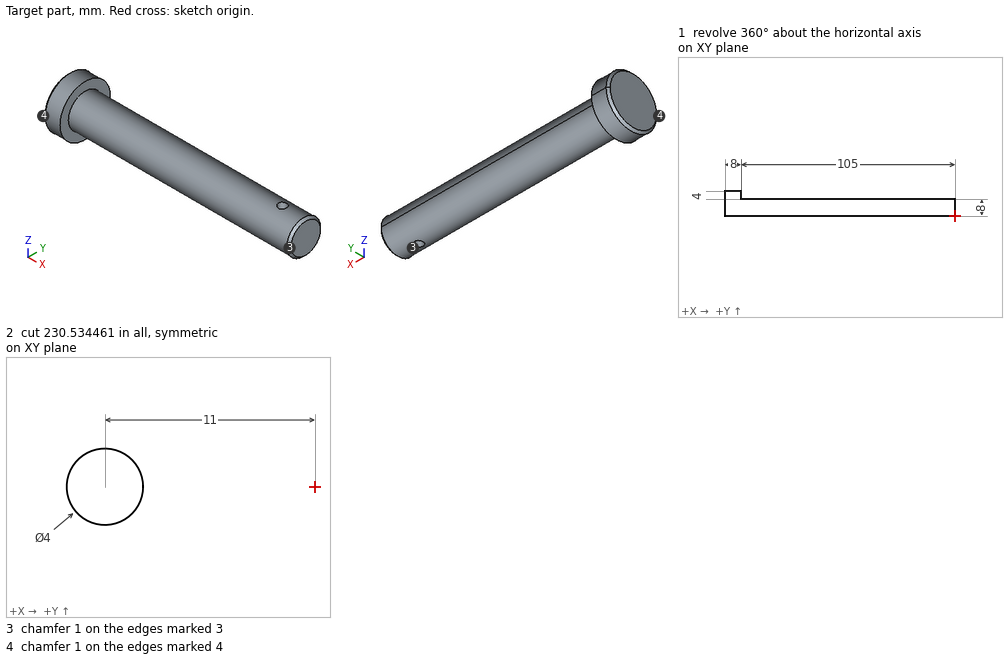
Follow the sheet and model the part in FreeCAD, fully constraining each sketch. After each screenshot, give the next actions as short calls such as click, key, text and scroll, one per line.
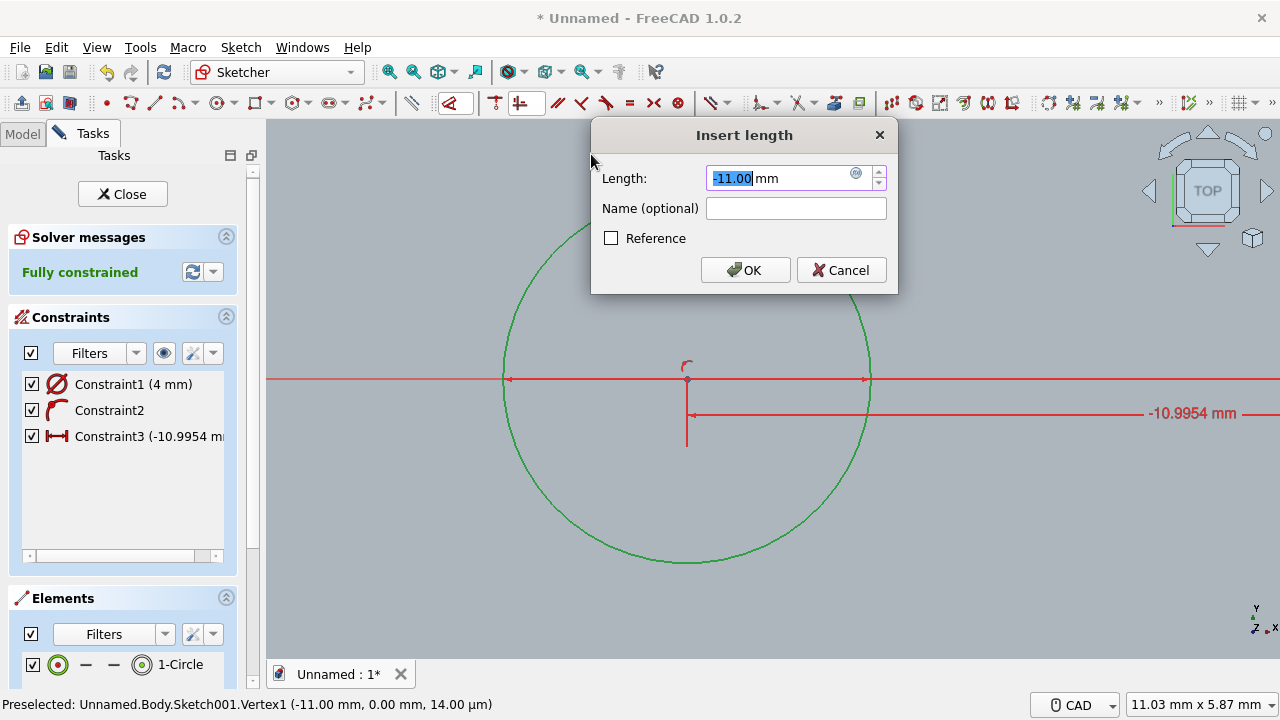
text(-11)
key(Return)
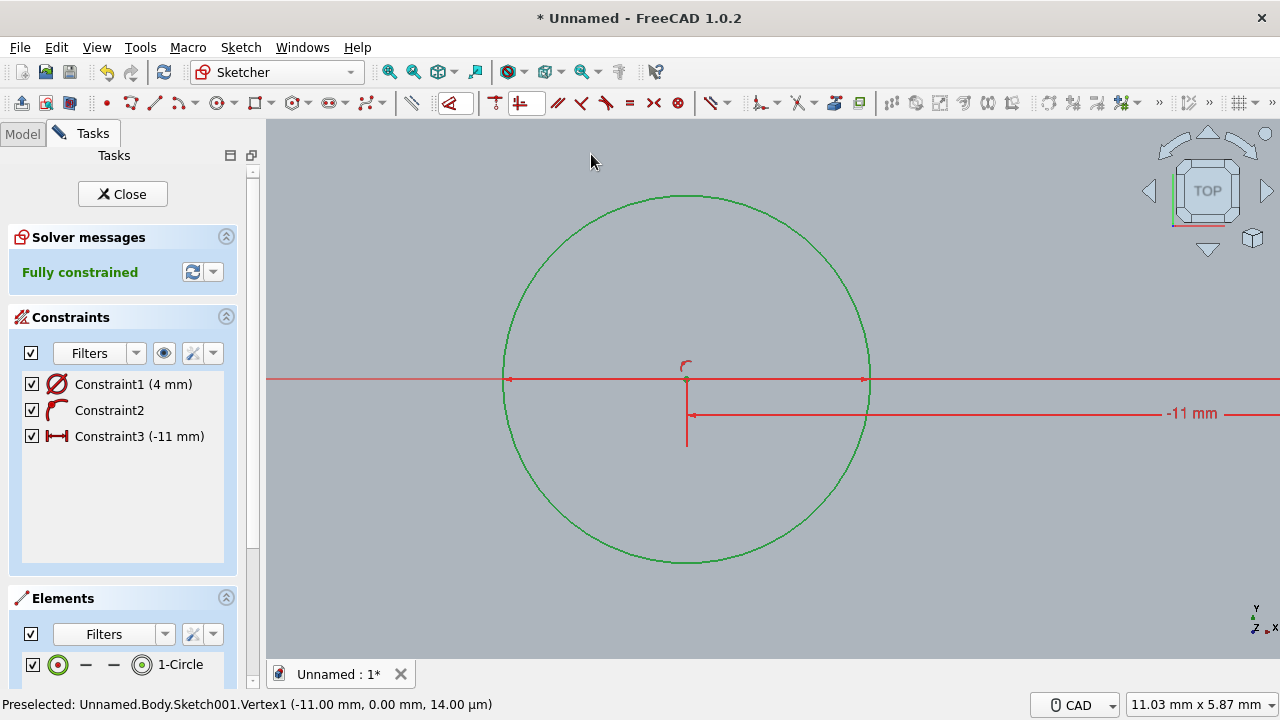
click(123, 194)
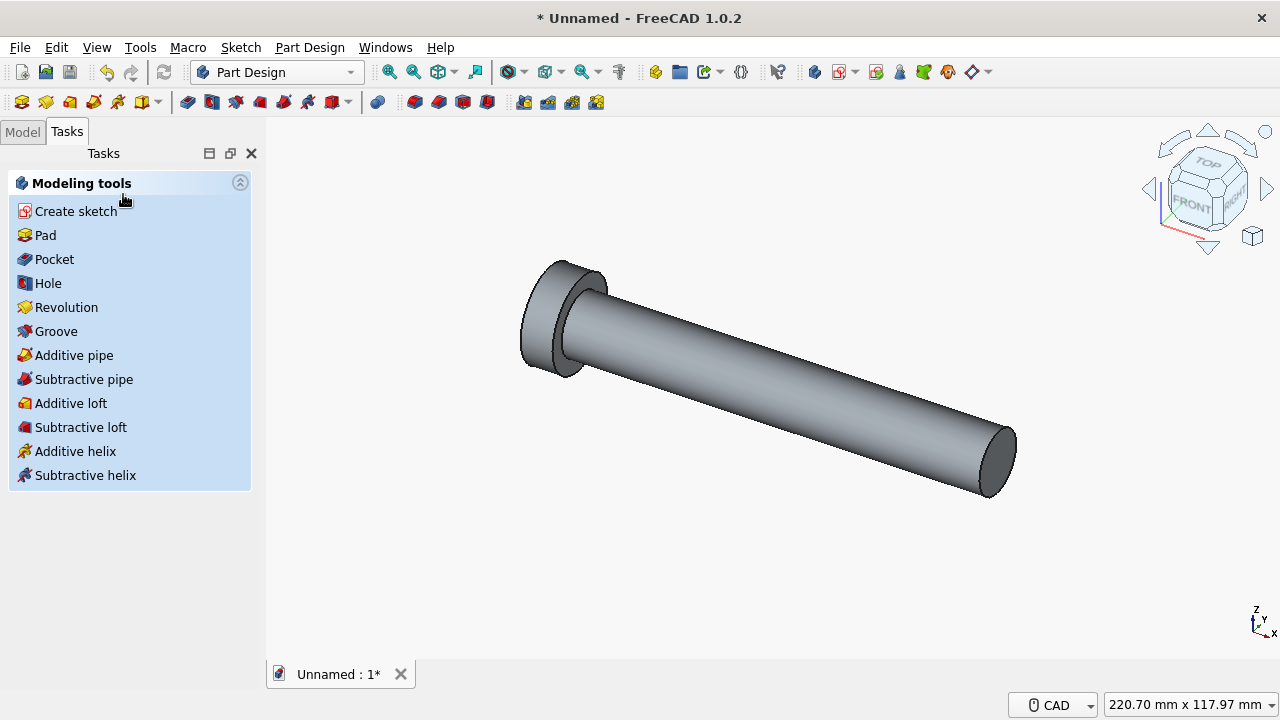
click(188, 102)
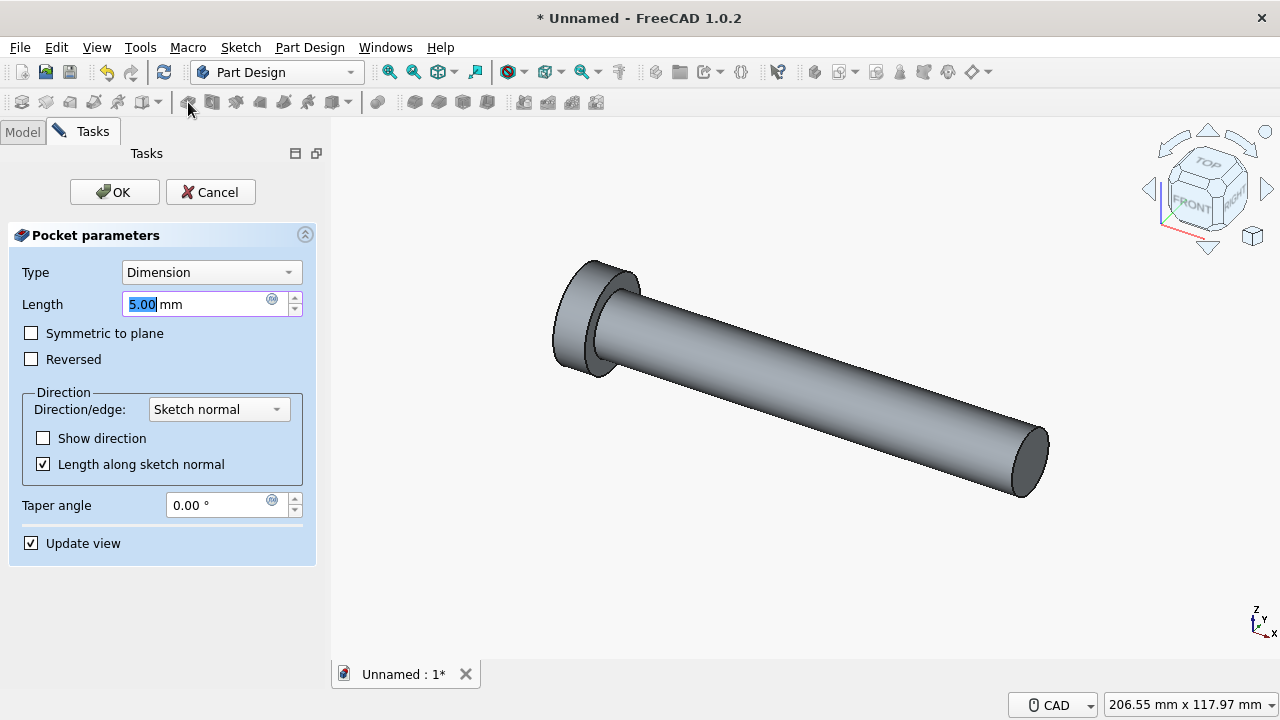
text(230.534461)
key(Tab)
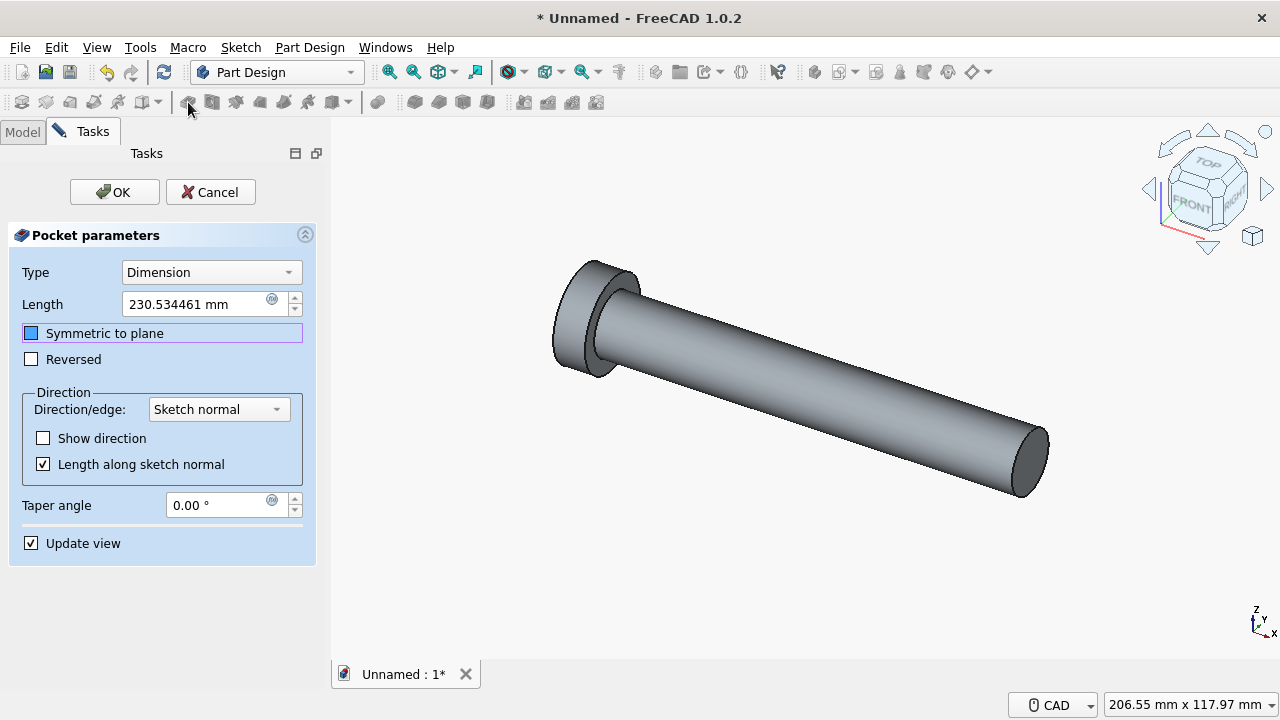
click(30, 333)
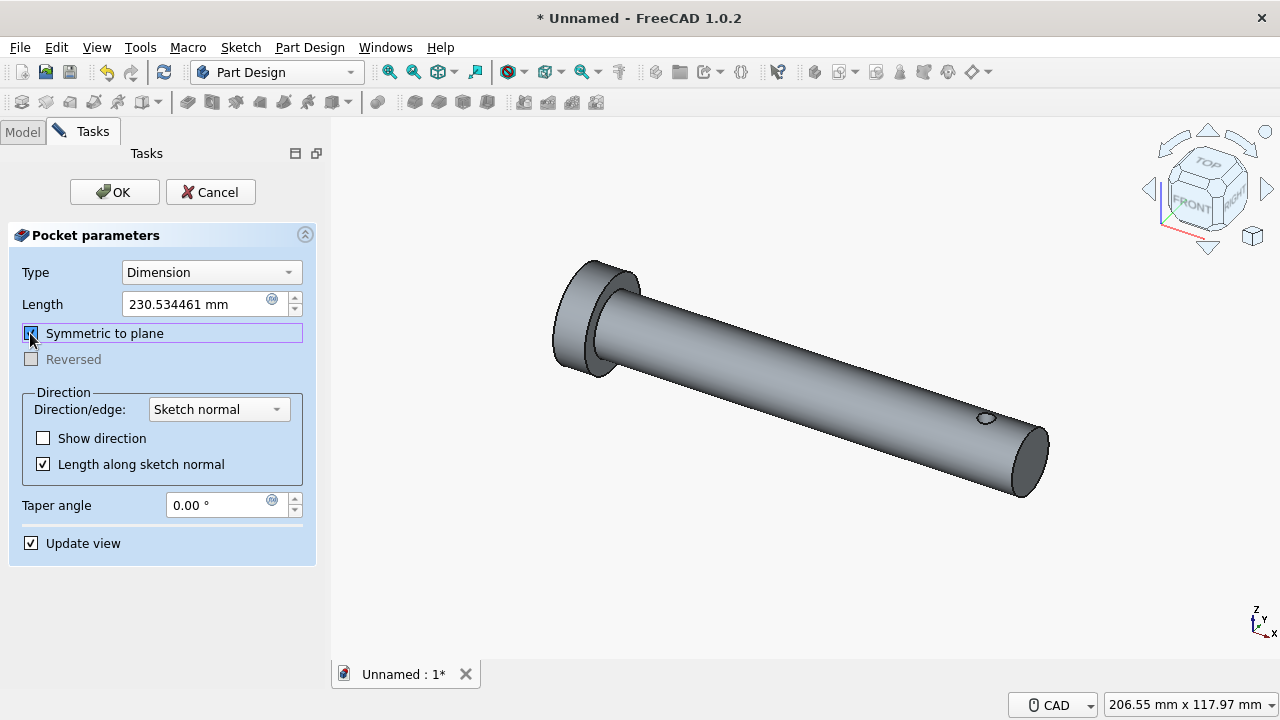
click(115, 192)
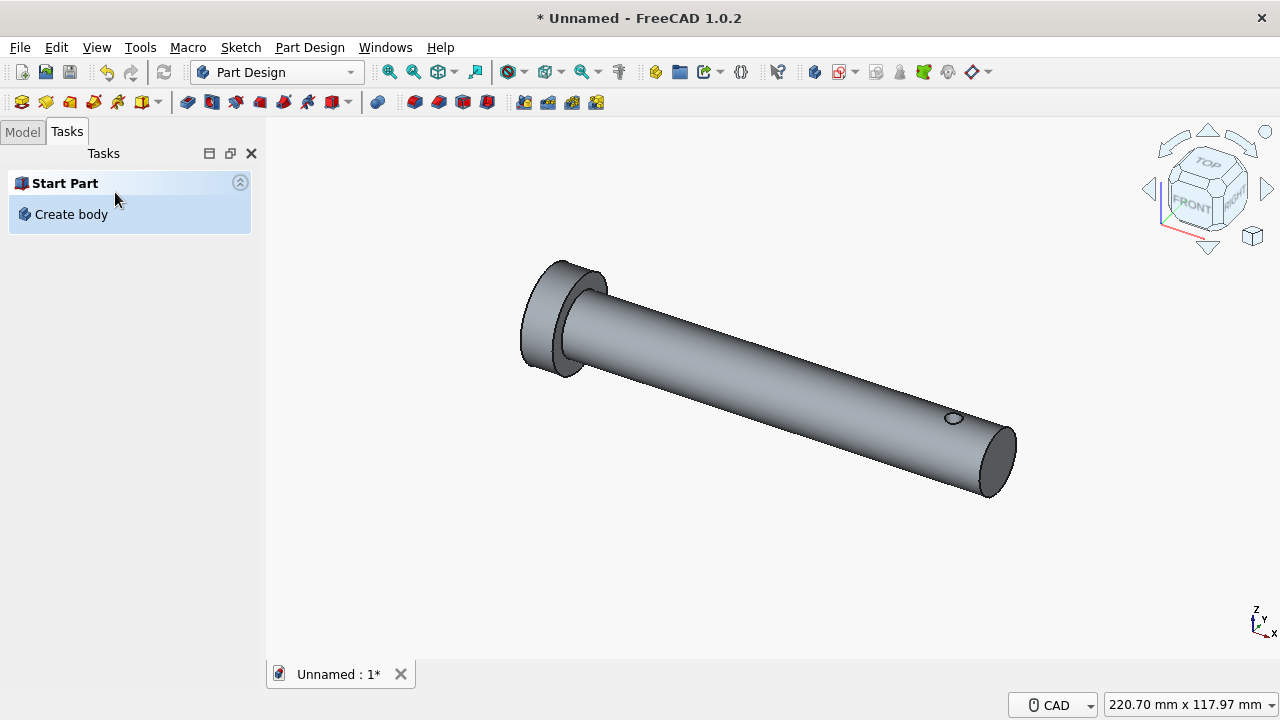
click(979, 480)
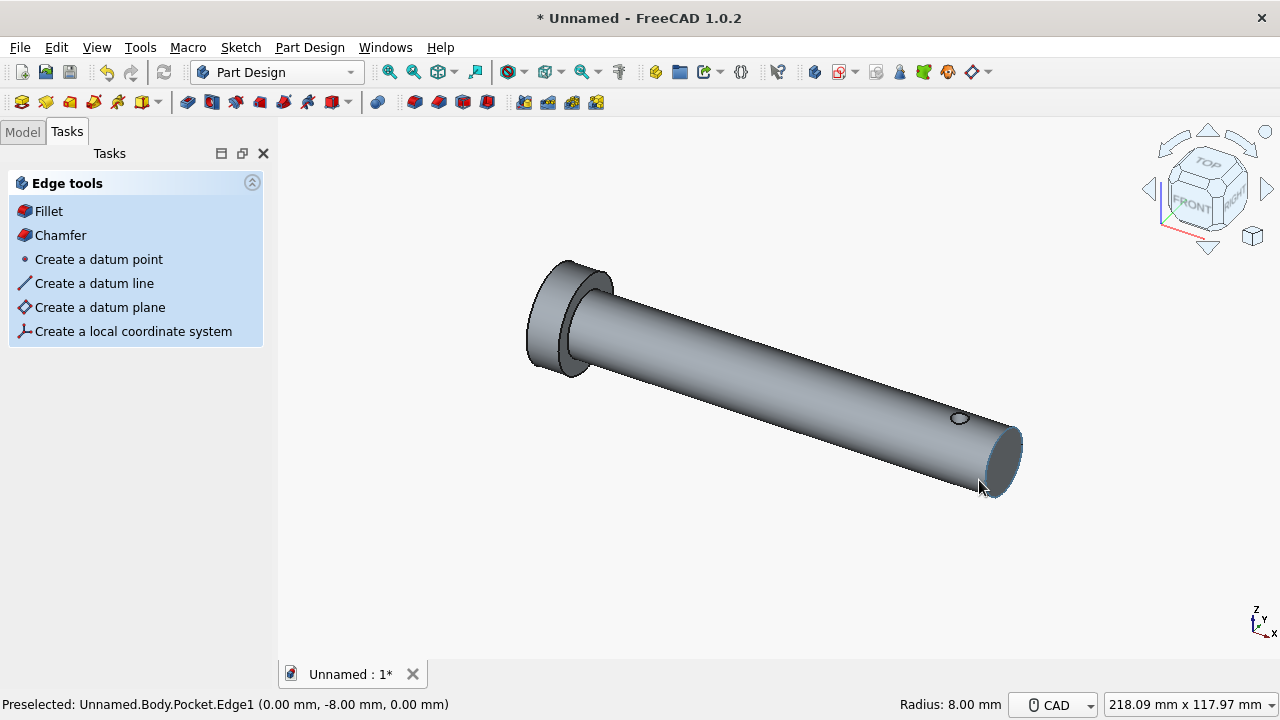
click(440, 102)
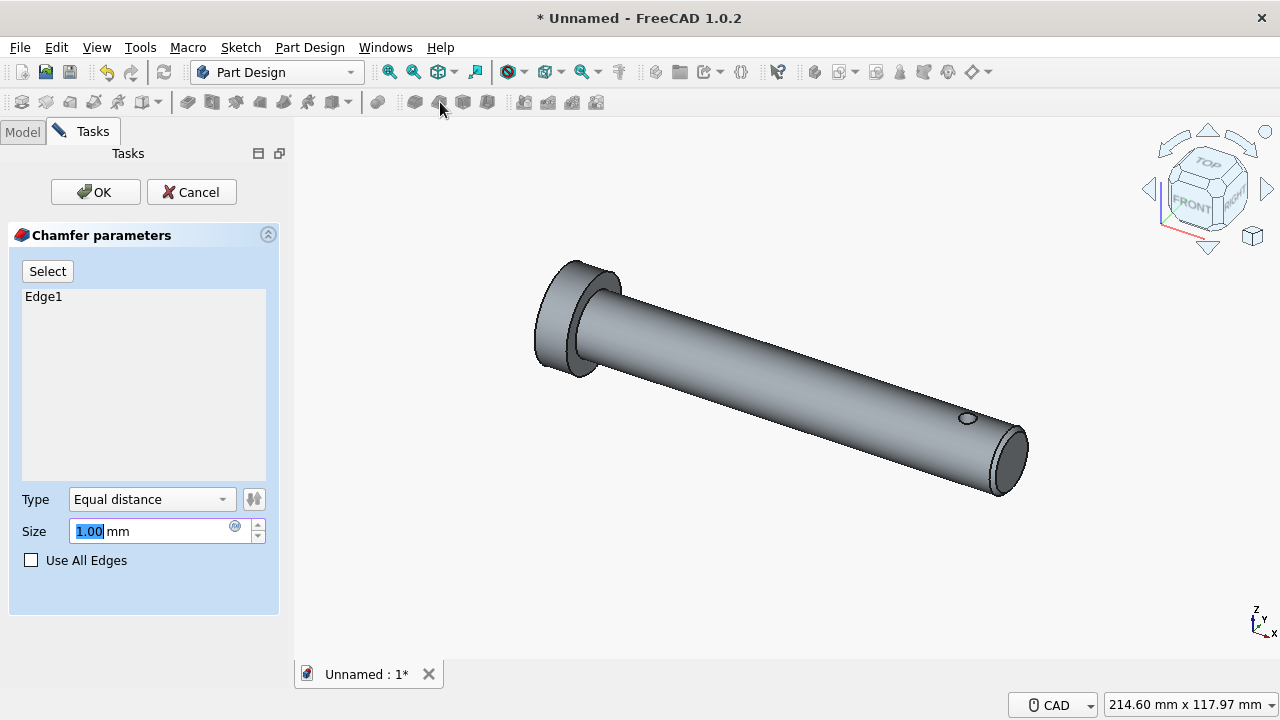
text(1)
key(Tab)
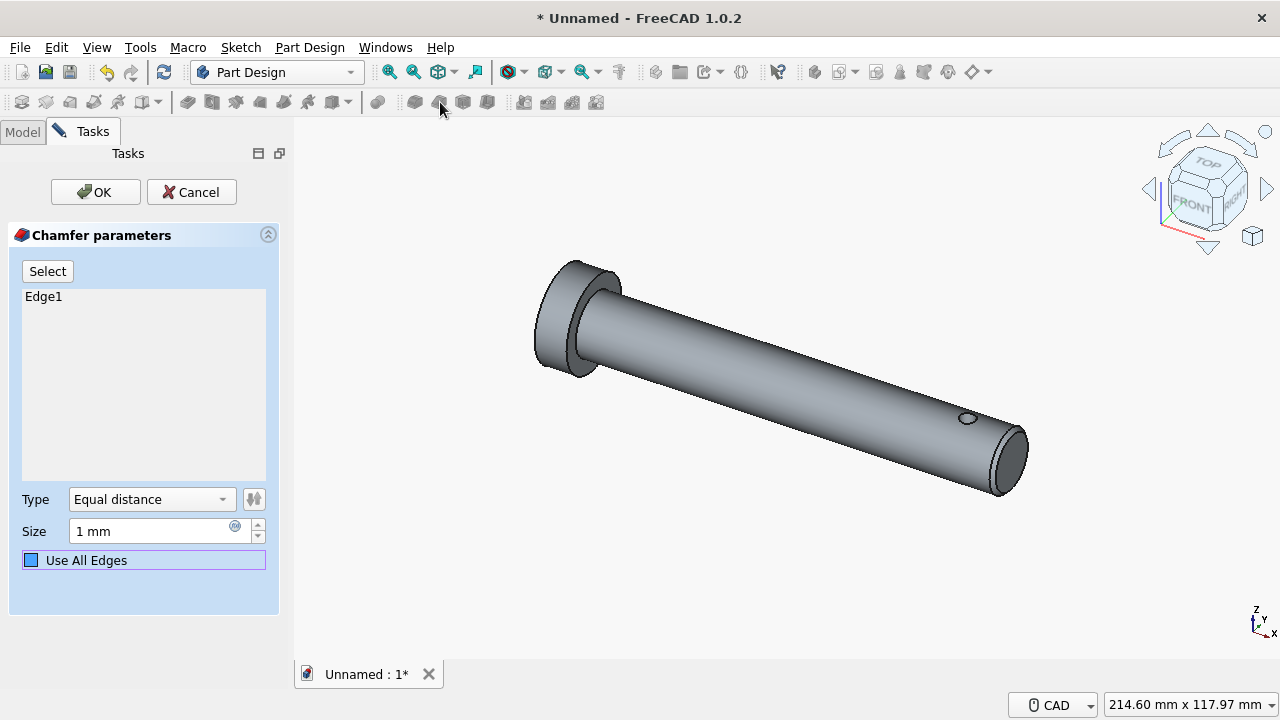
click(96, 192)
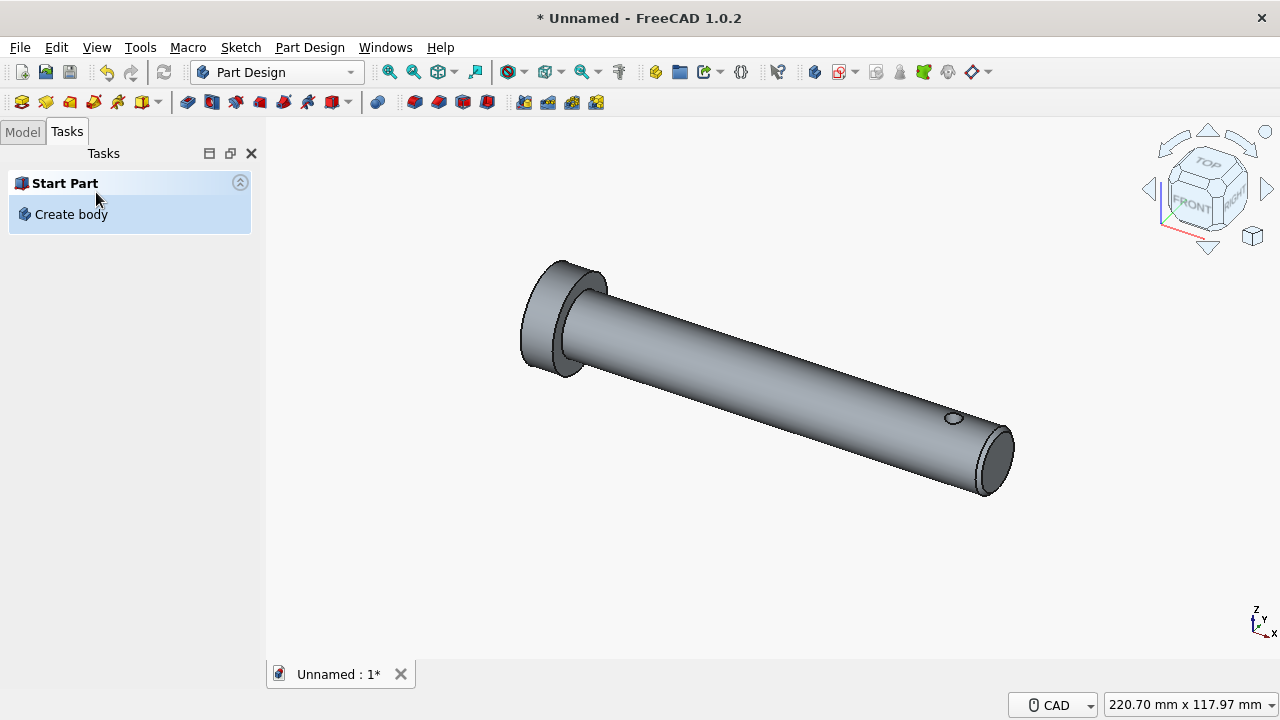
key(0)